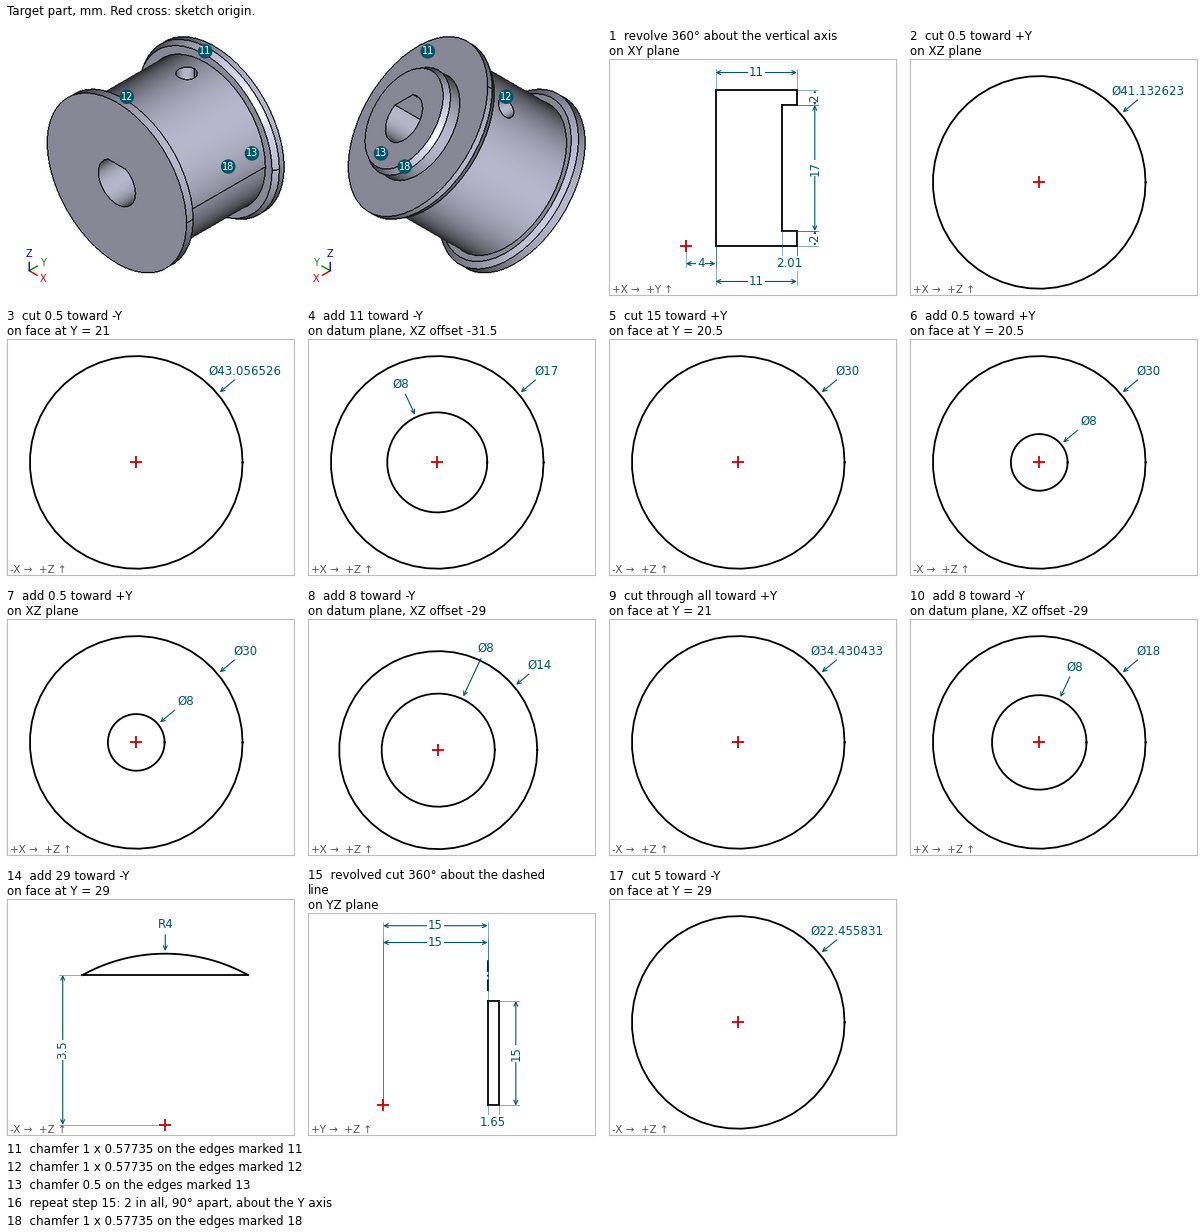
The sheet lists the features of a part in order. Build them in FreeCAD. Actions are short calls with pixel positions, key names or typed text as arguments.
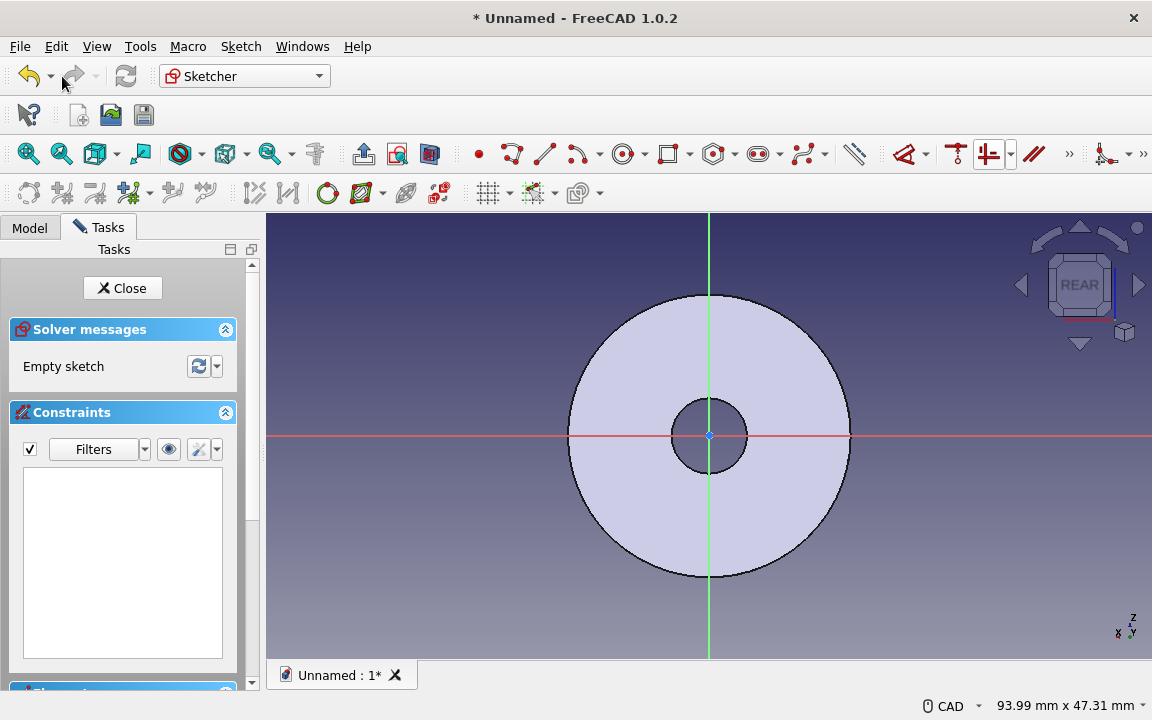
click(622, 154)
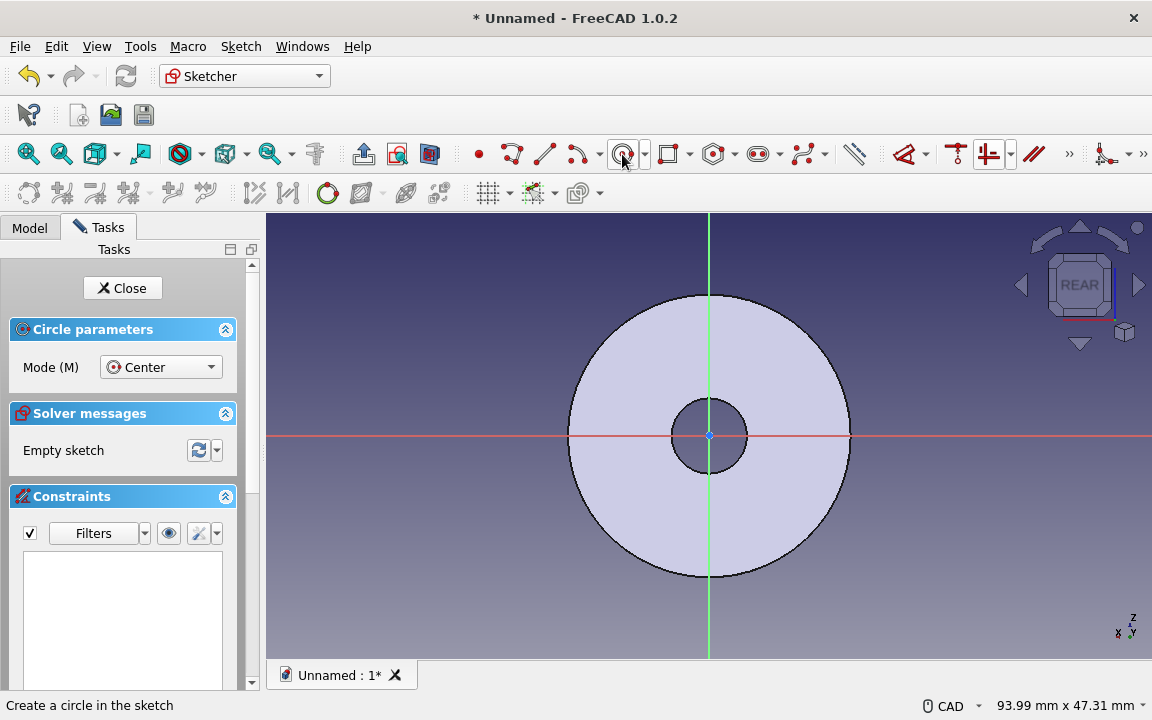
click(709, 436)
move(809, 336)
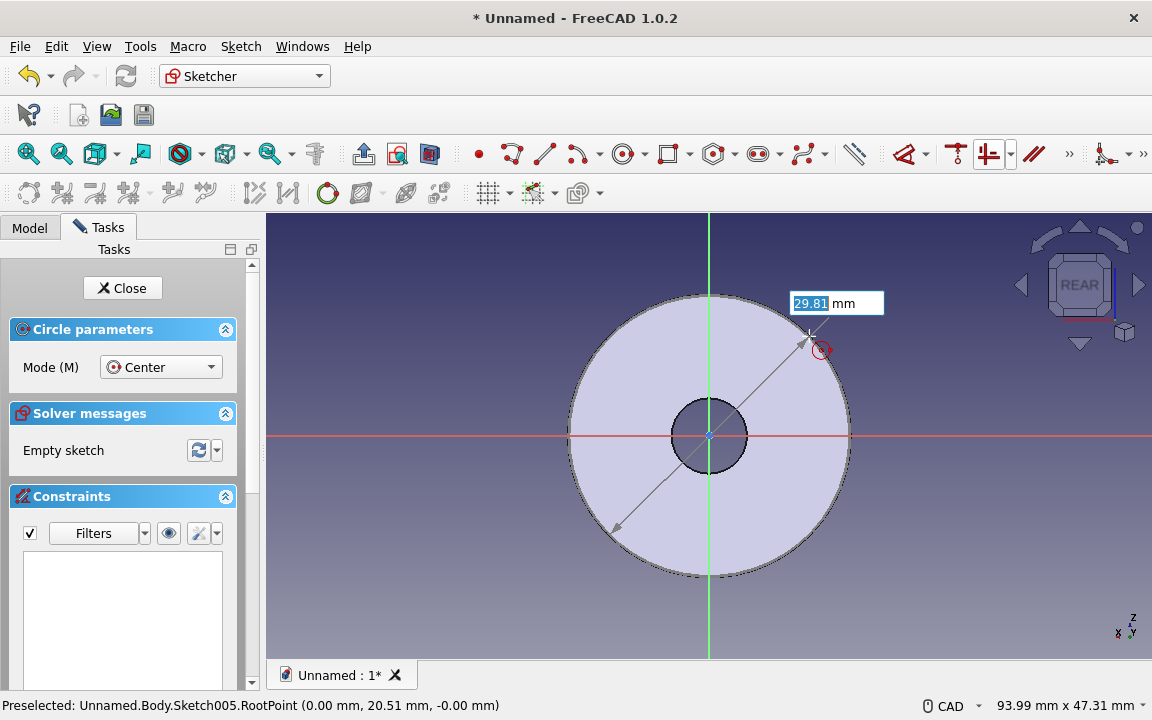
text(30)
key(Return)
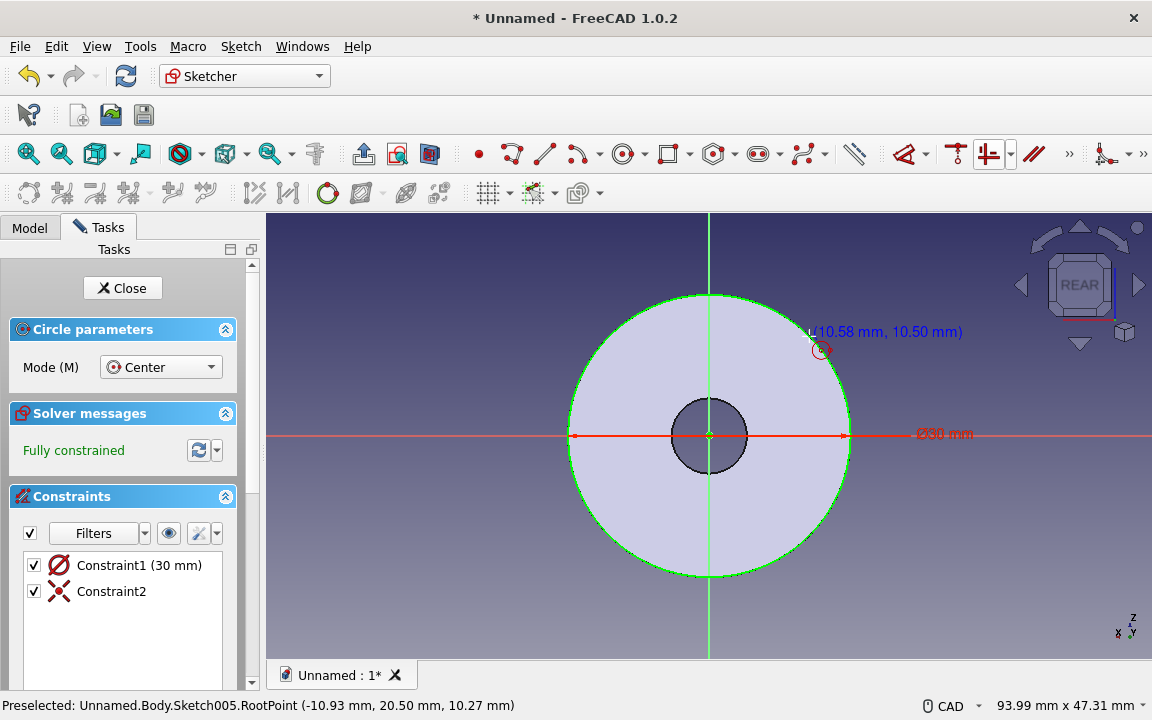
click(709, 436)
move(736, 409)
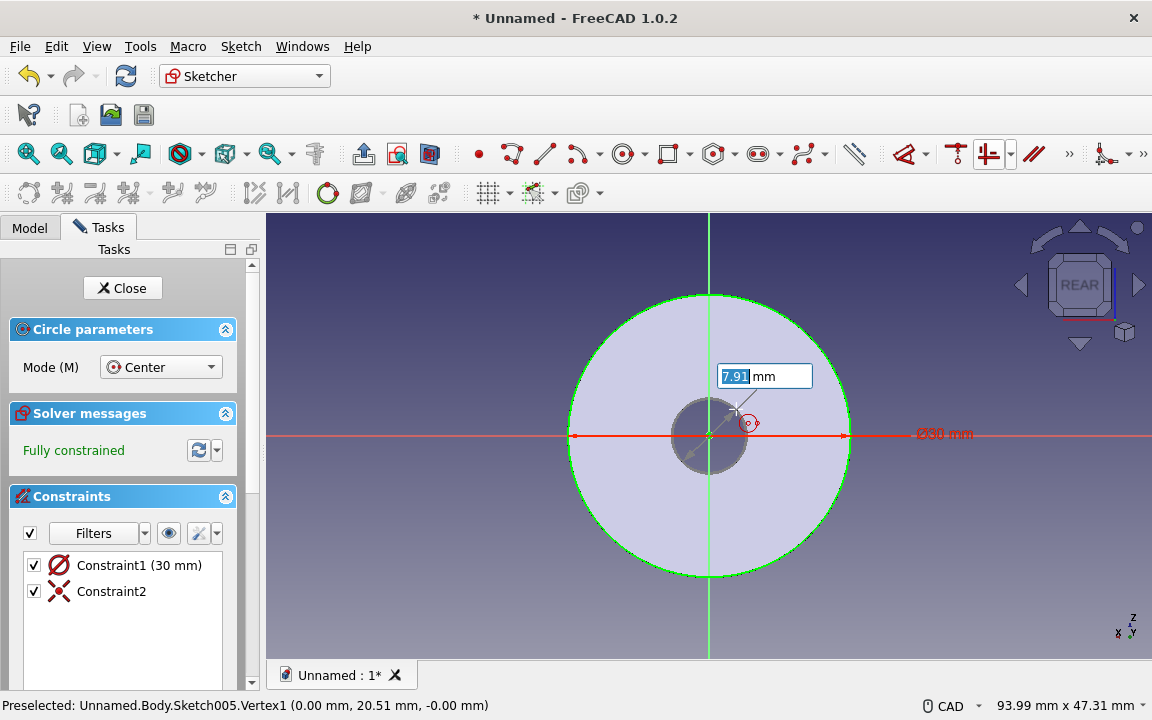
text(8)
key(Return)
key(Escape)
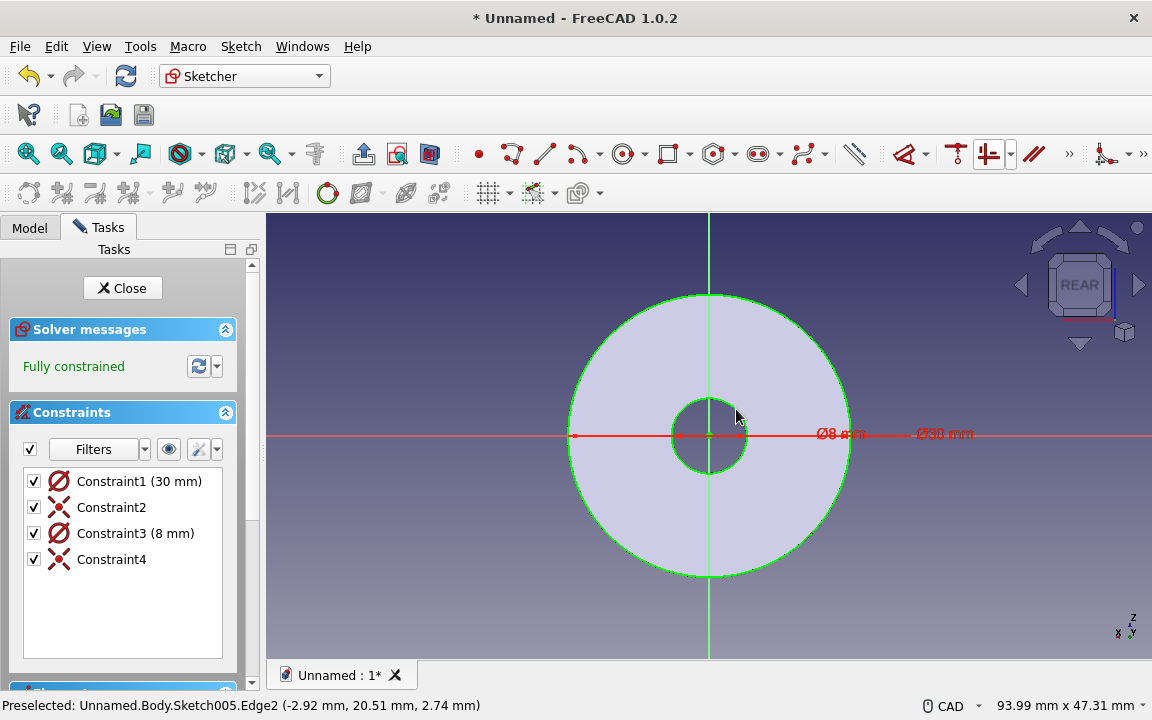
click(123, 288)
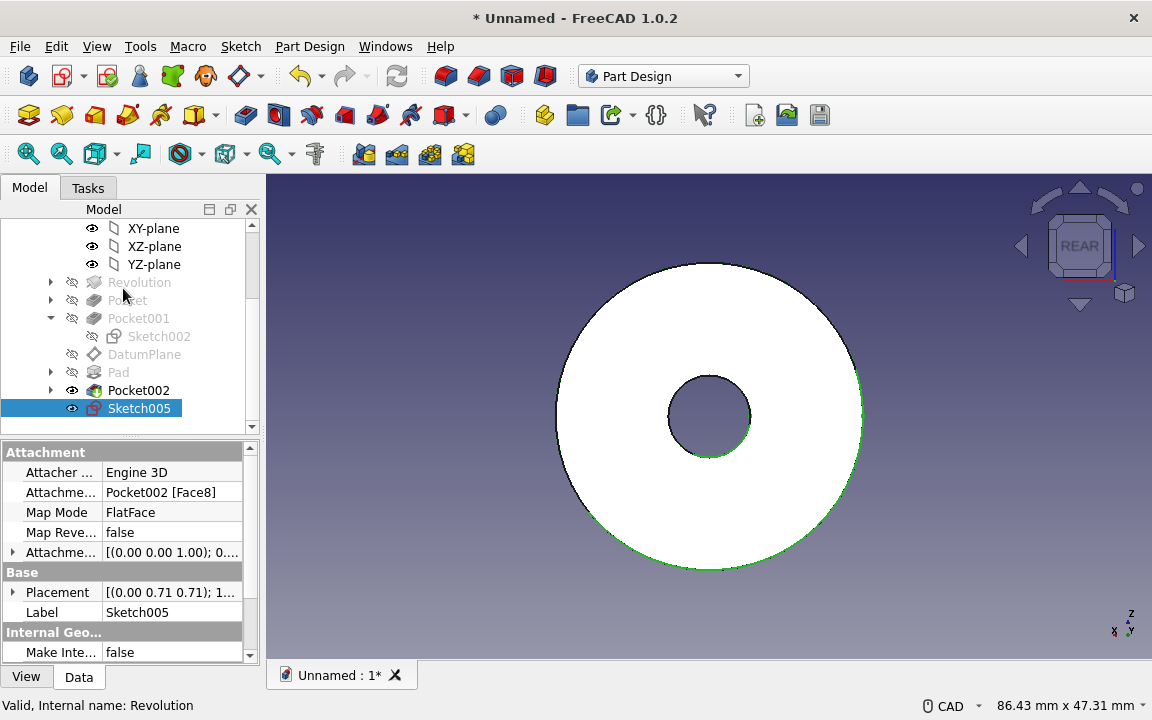
click(29, 116)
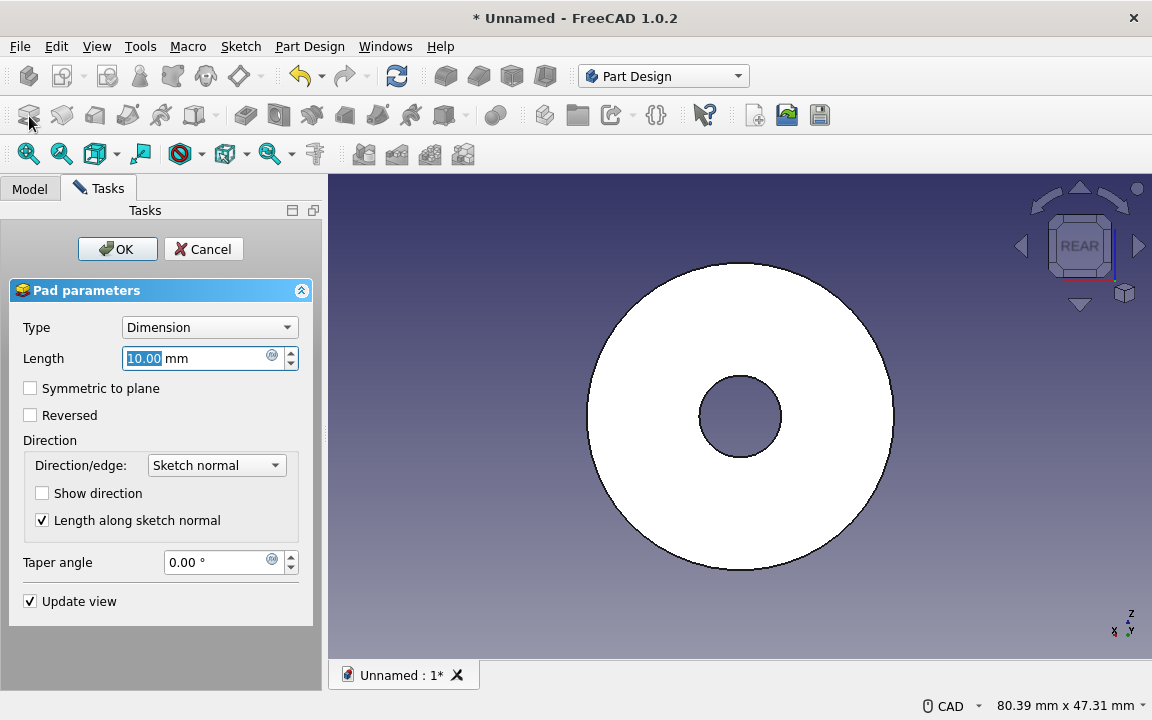
text(0.5)
key(Tab)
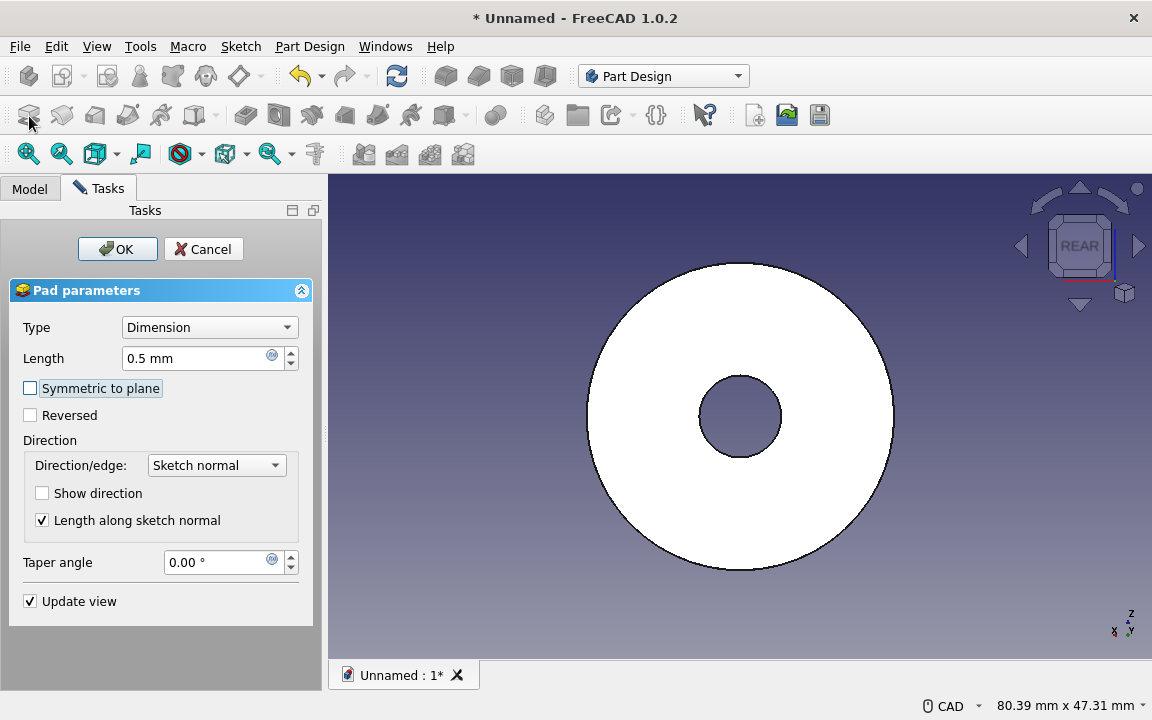
click(118, 249)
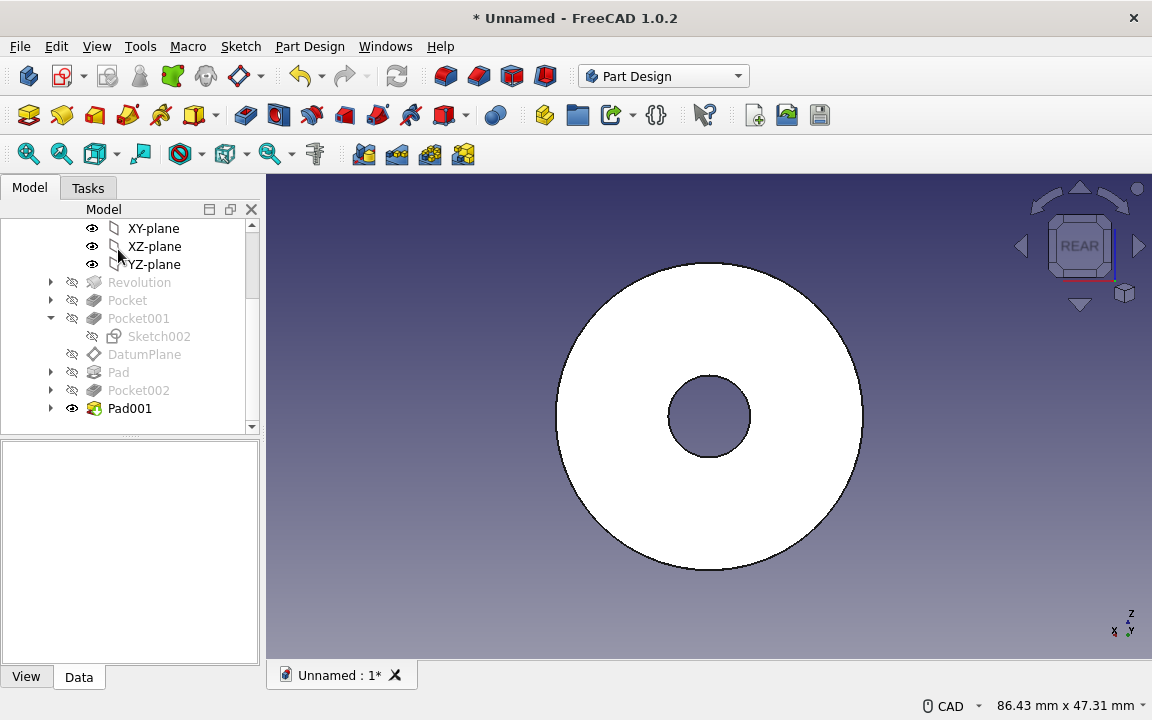
click(62, 76)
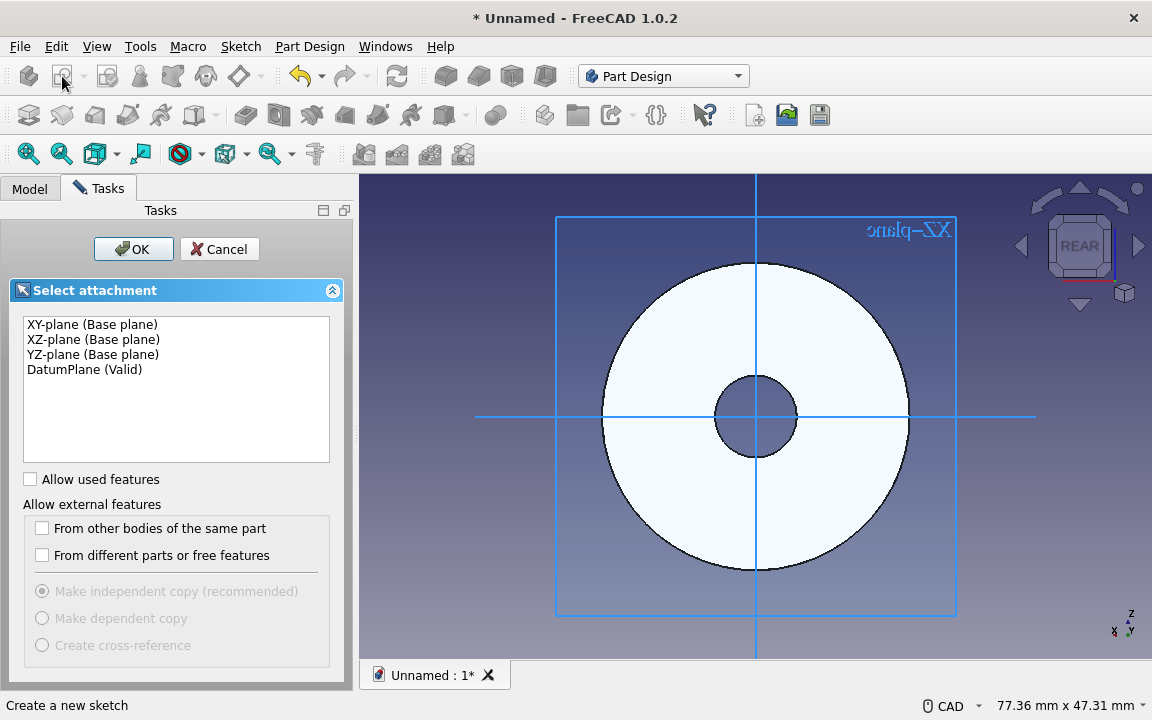
click(84, 340)